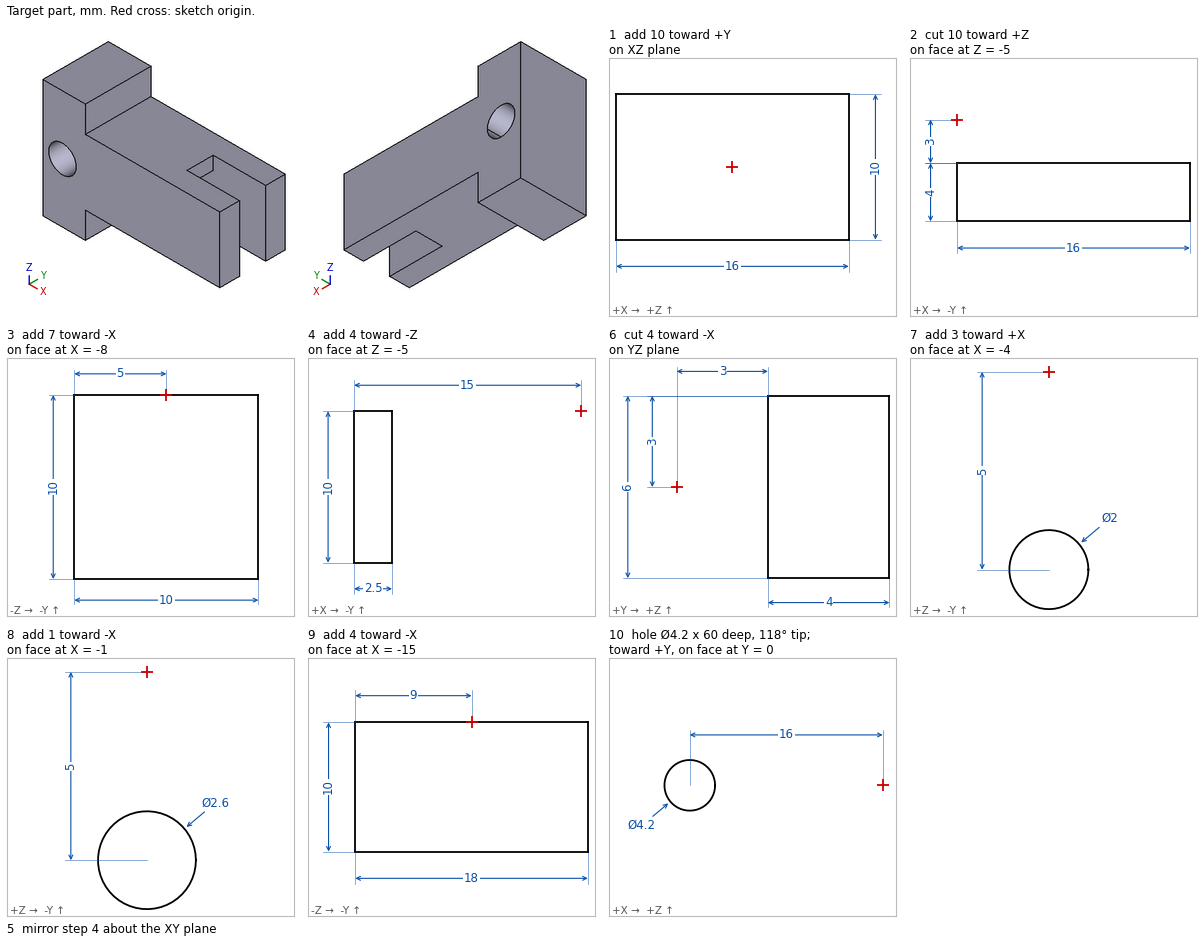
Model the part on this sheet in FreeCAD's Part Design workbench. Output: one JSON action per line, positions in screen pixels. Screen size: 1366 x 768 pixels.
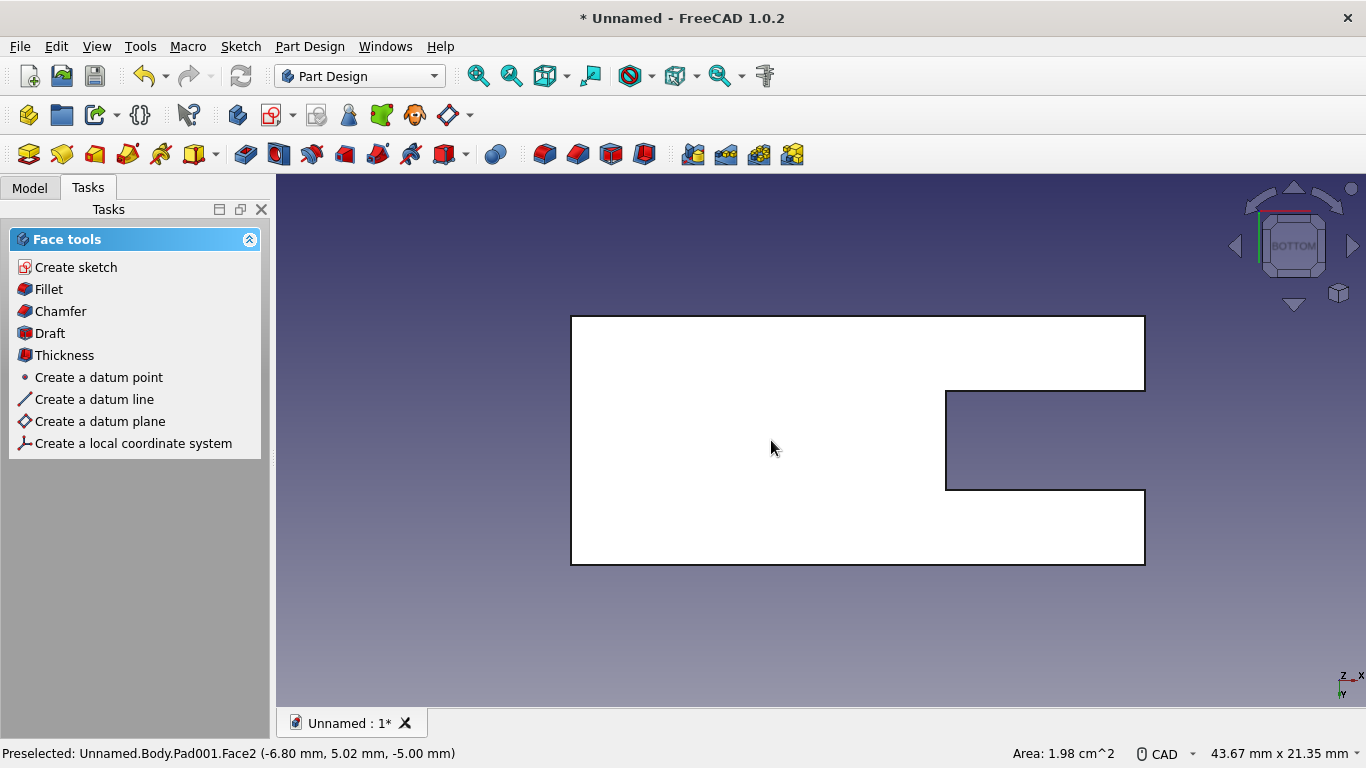
{"action": "left_click", "coordinate": [270, 116]}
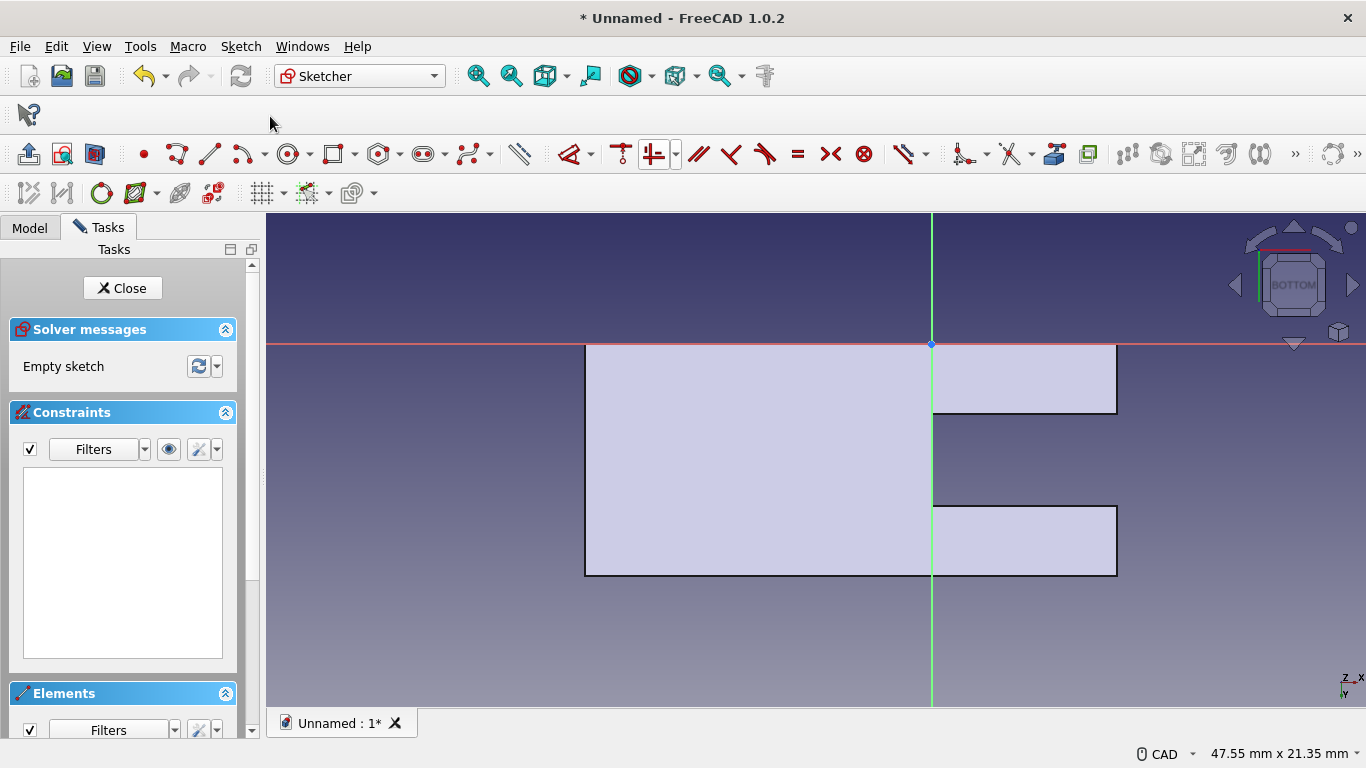
{"action": "left_click", "coordinate": [332, 154]}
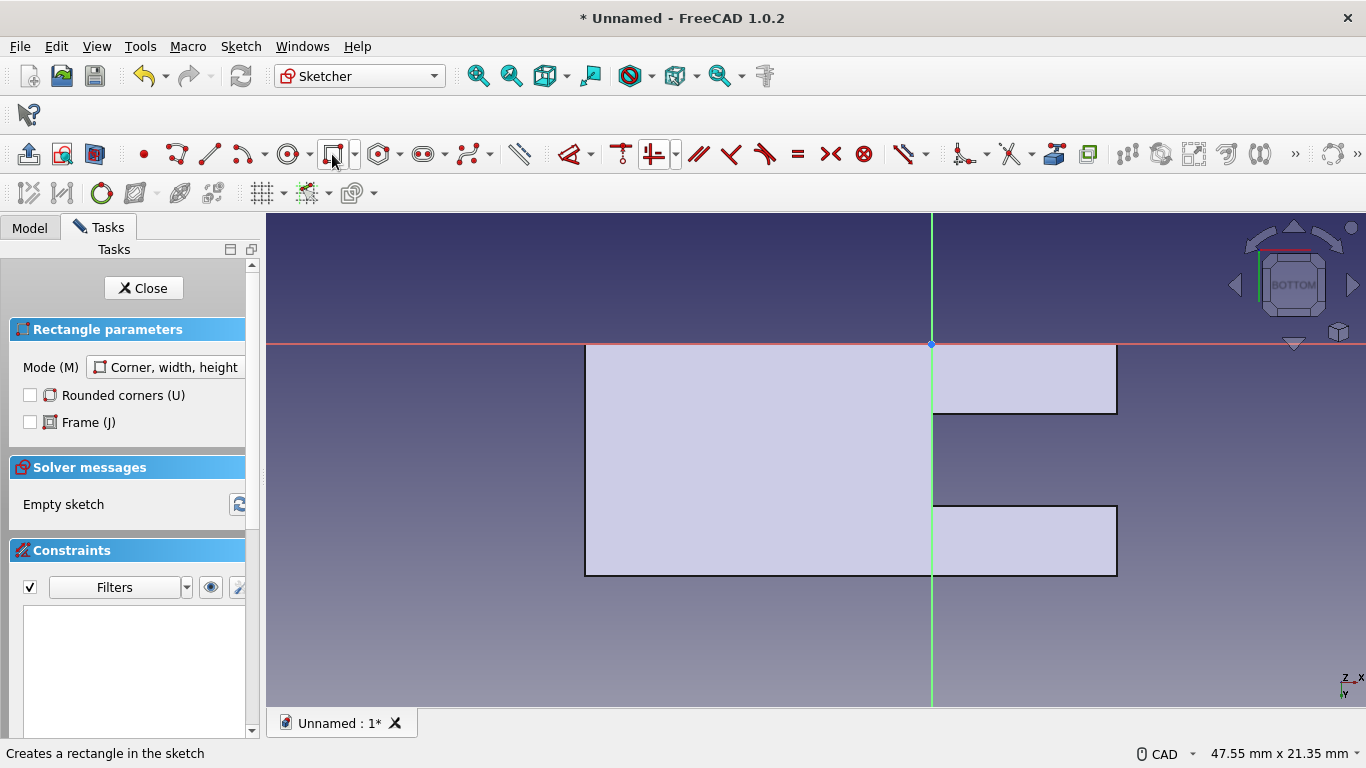
{"action": "left_click", "coordinate": [585, 344]}
{"action": "left_click", "coordinate": [642, 576]}
{"action": "key", "text": "Escape"}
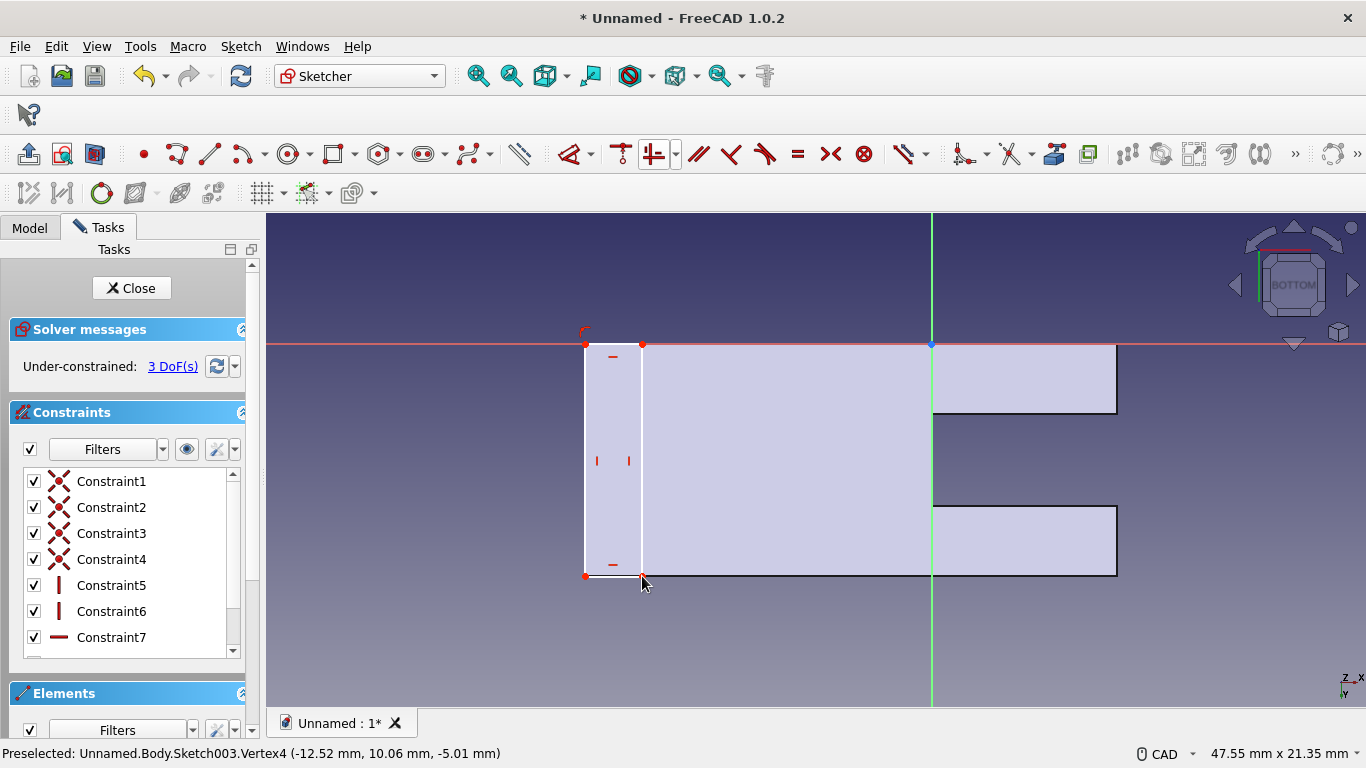
{"action": "left_click", "coordinate": [568, 154]}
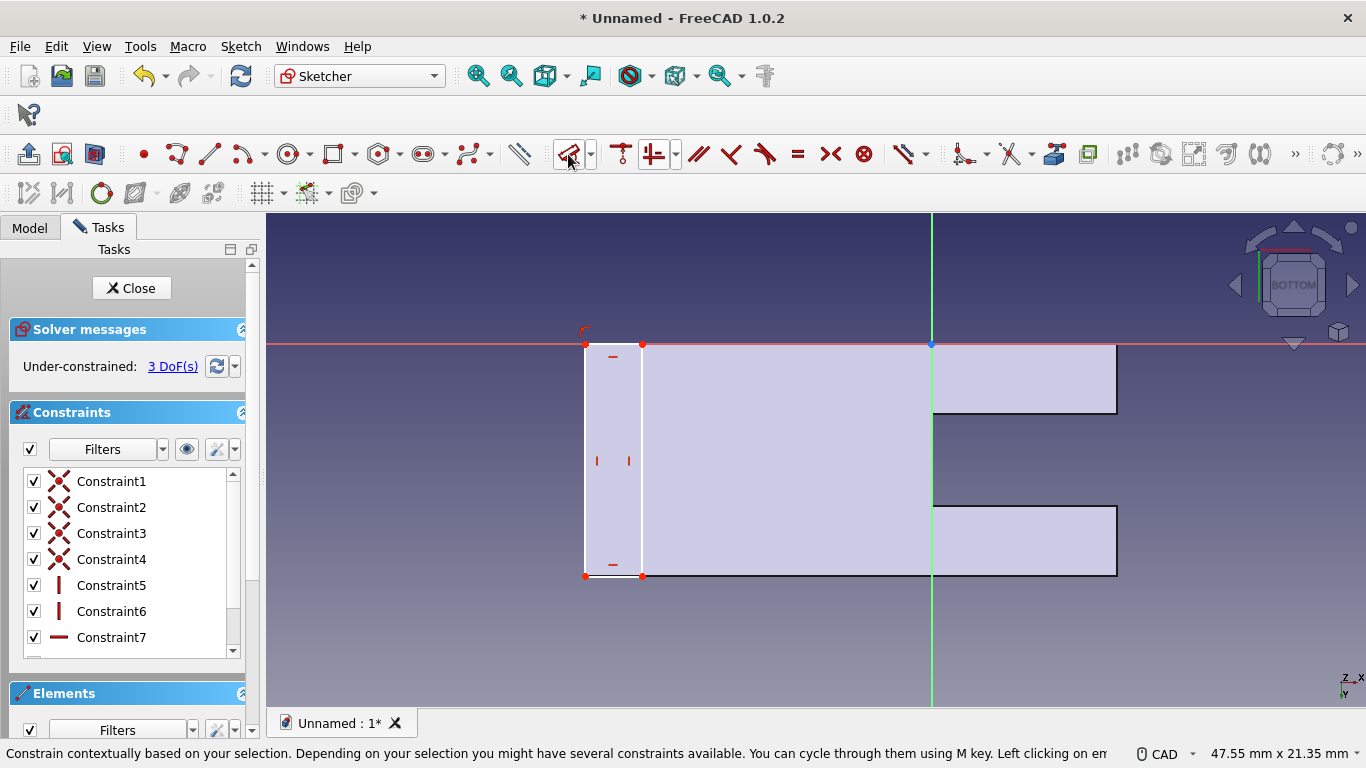
{"action": "left_click", "coordinate": [585, 414]}
{"action": "left_click", "coordinate": [551, 461]}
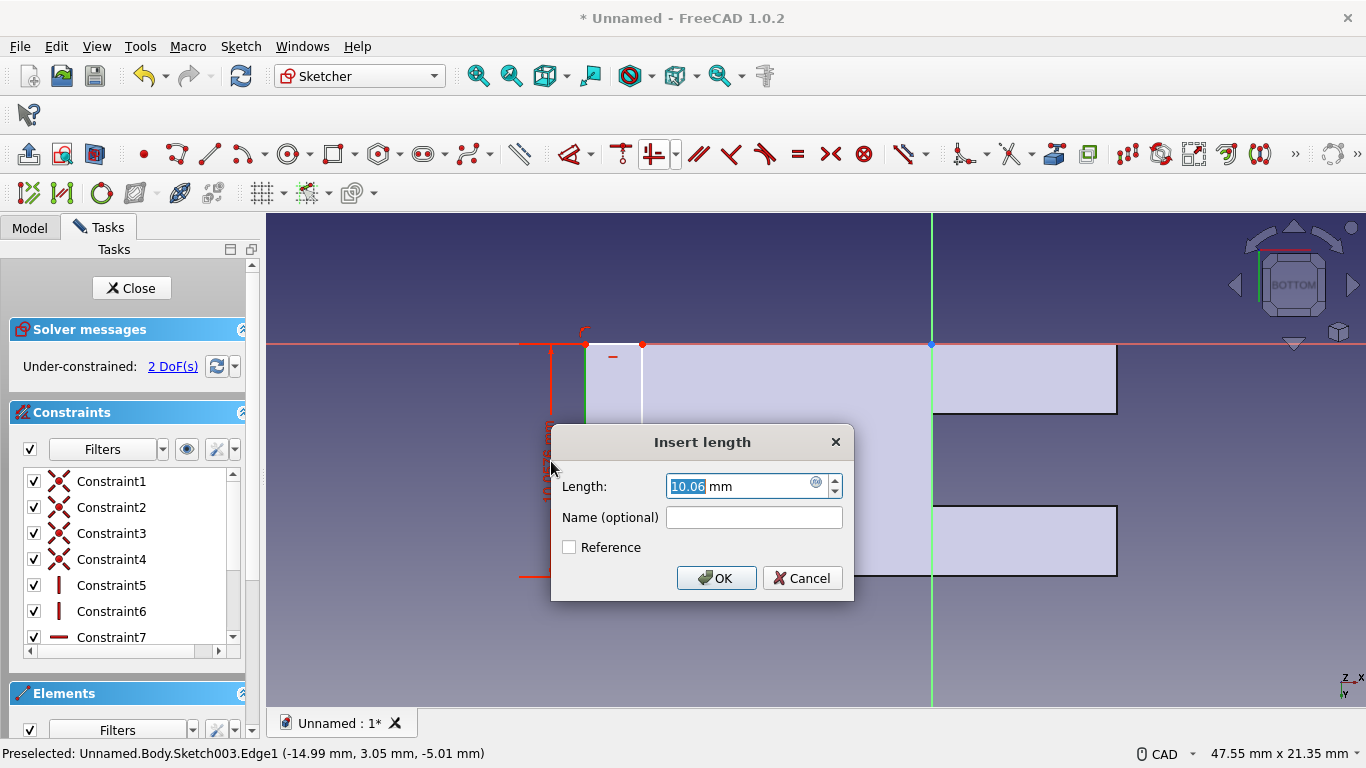
{"action": "type", "text": "10"}
{"action": "key", "text": "Return"}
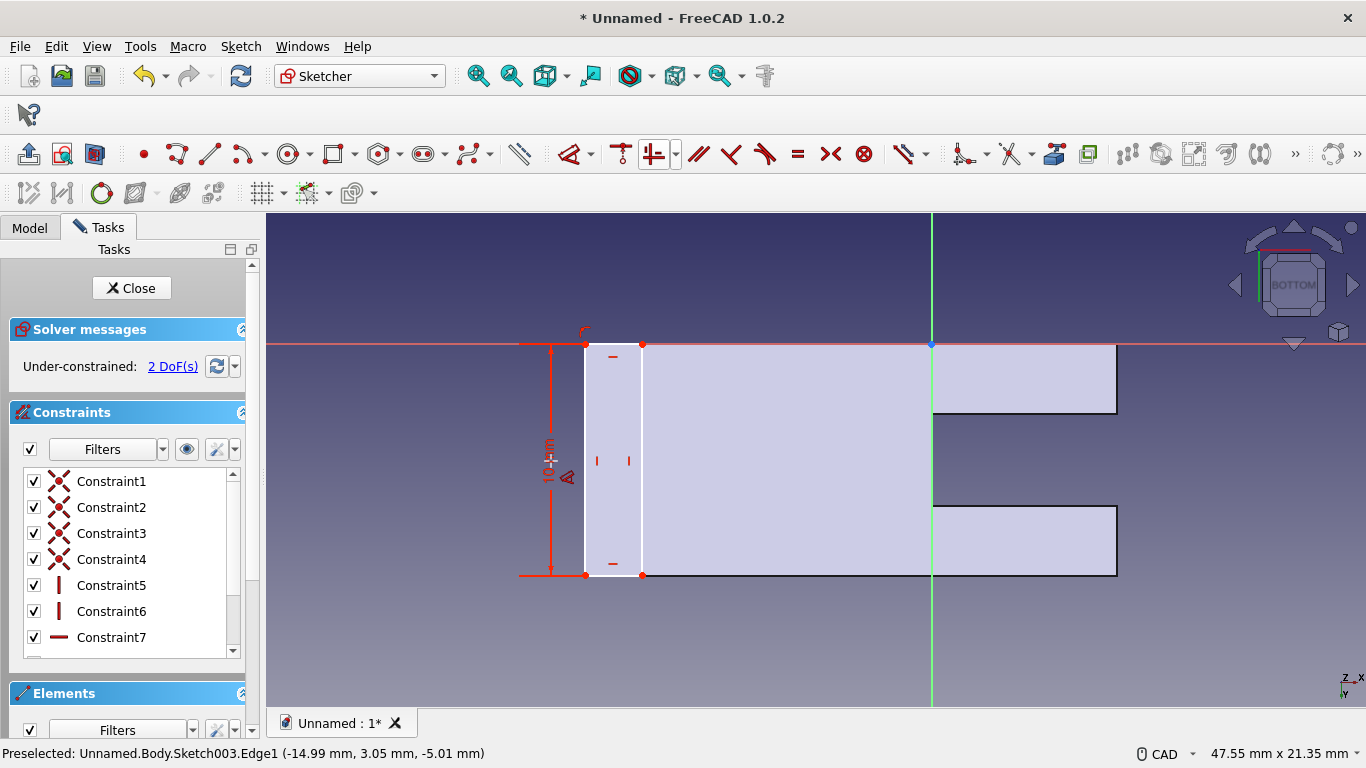
{"action": "left_click", "coordinate": [602, 576]}
{"action": "left_click", "coordinate": [614, 610]}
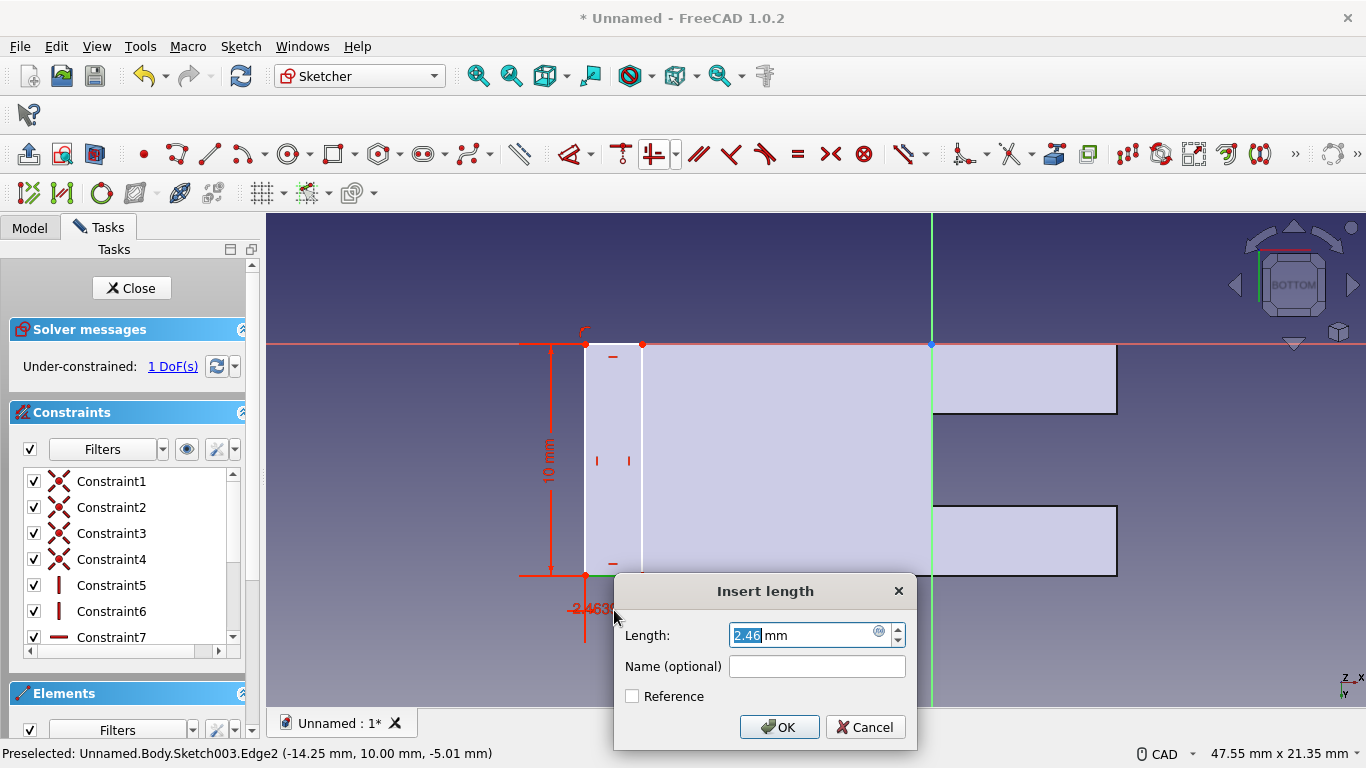
{"action": "type", "text": "2.5"}
{"action": "key", "text": "Return"}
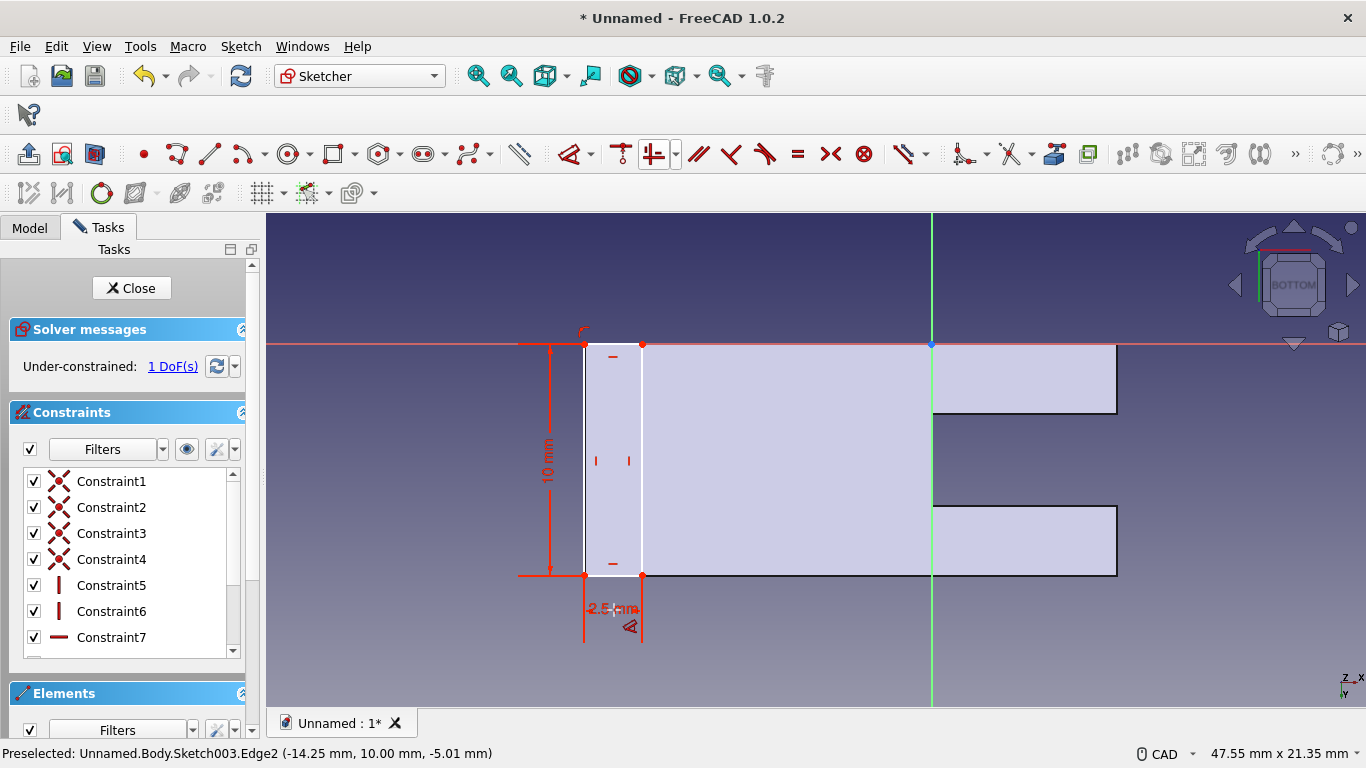
{"action": "left_click", "coordinate": [584, 344]}
{"action": "left_click", "coordinate": [758, 310]}